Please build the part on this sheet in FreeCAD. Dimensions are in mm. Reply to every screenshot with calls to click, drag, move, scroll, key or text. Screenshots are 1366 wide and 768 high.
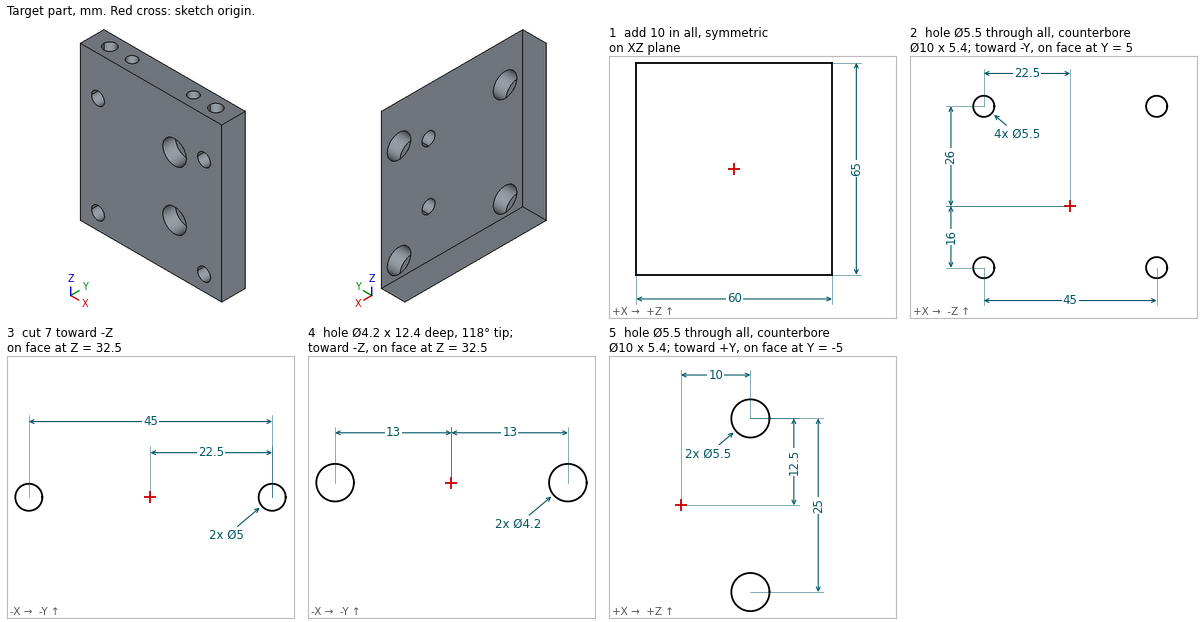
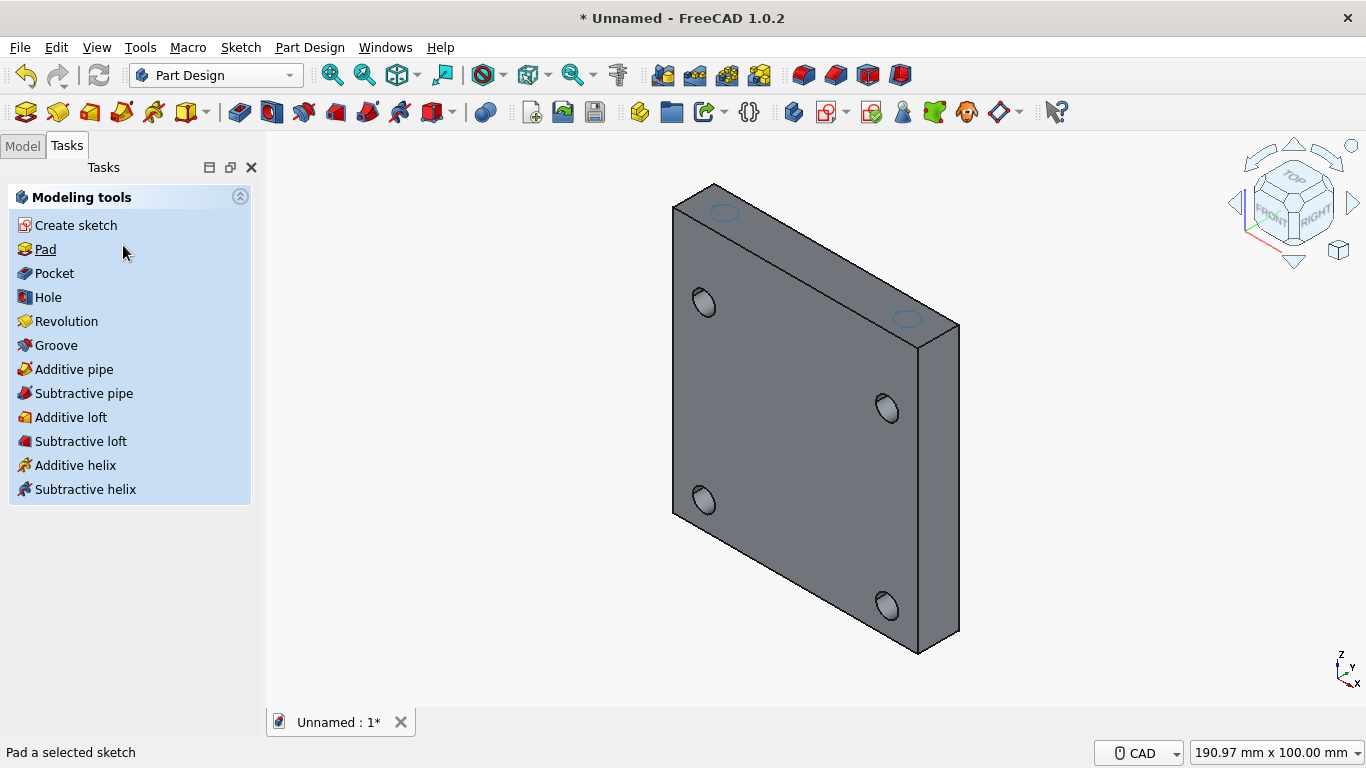
click(240, 112)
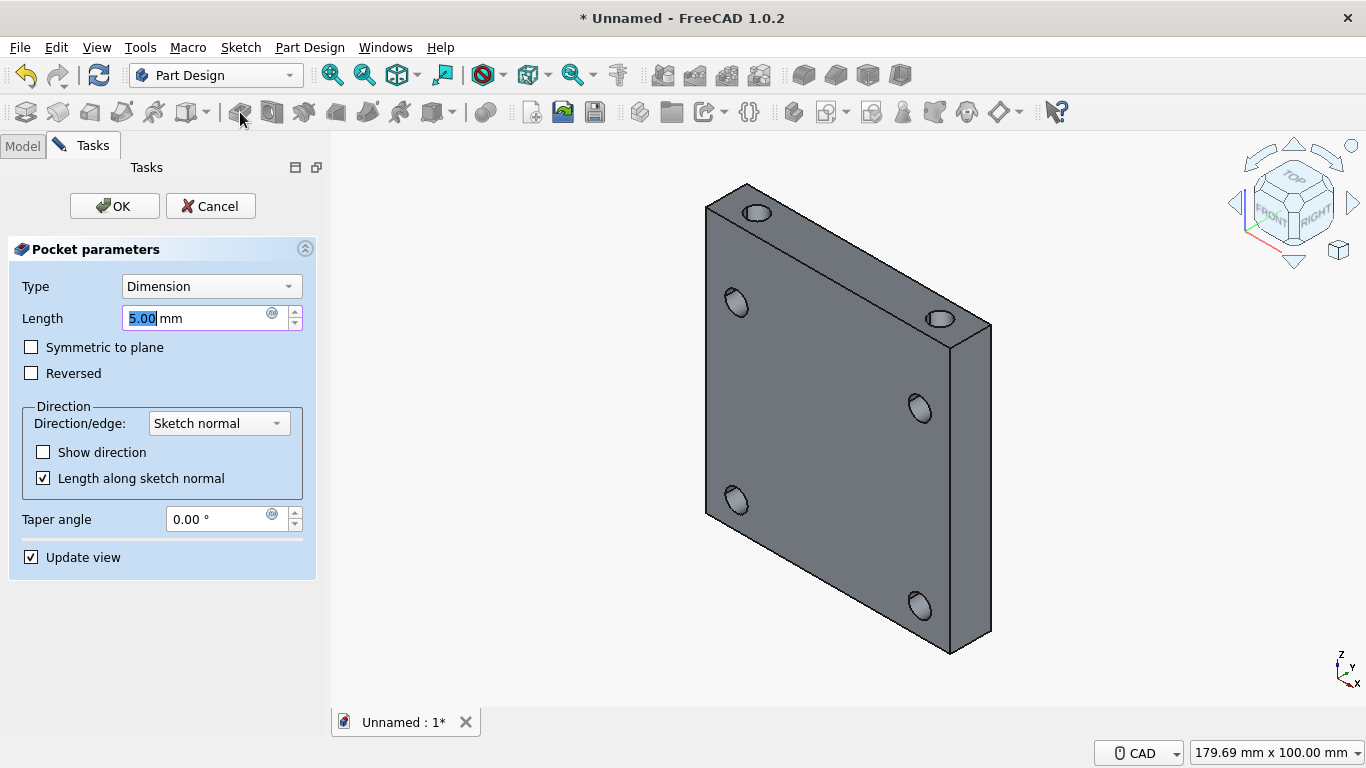
text(7)
key(Tab)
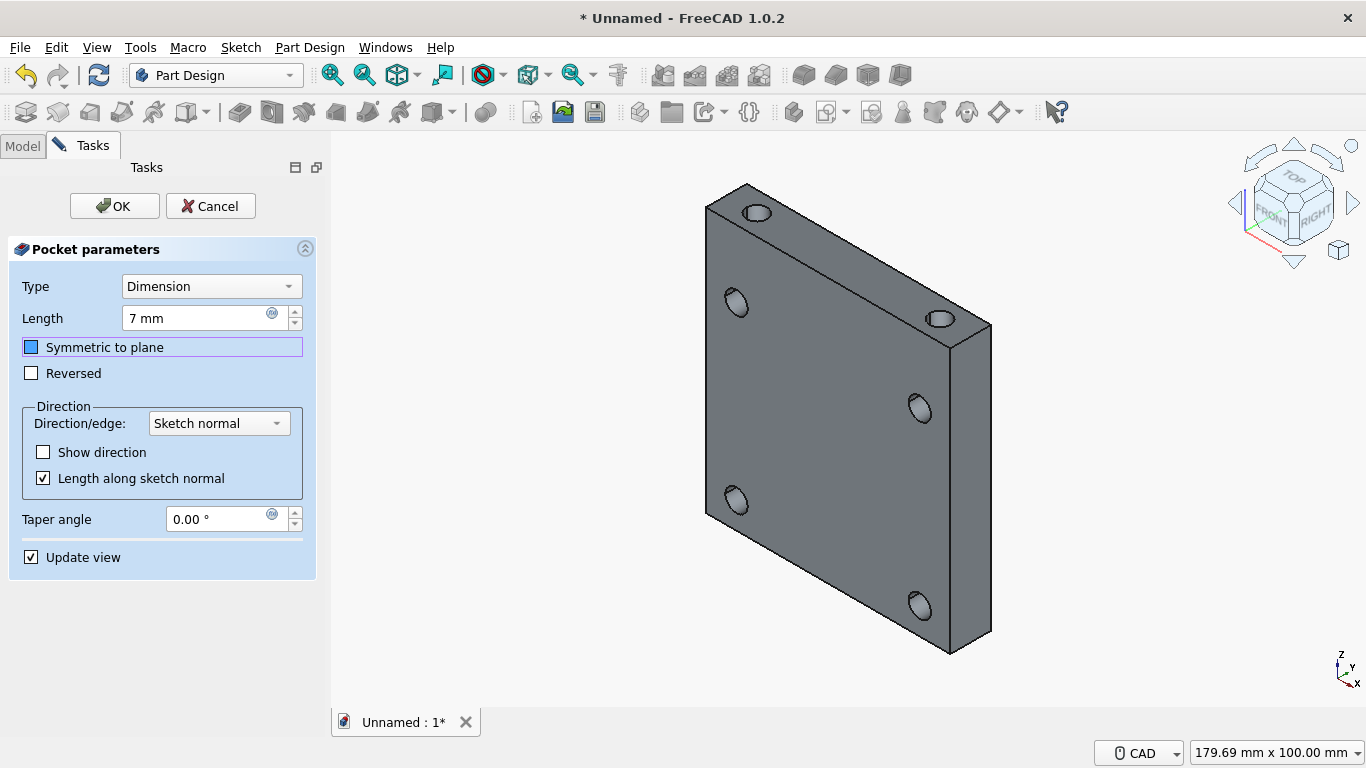
click(115, 206)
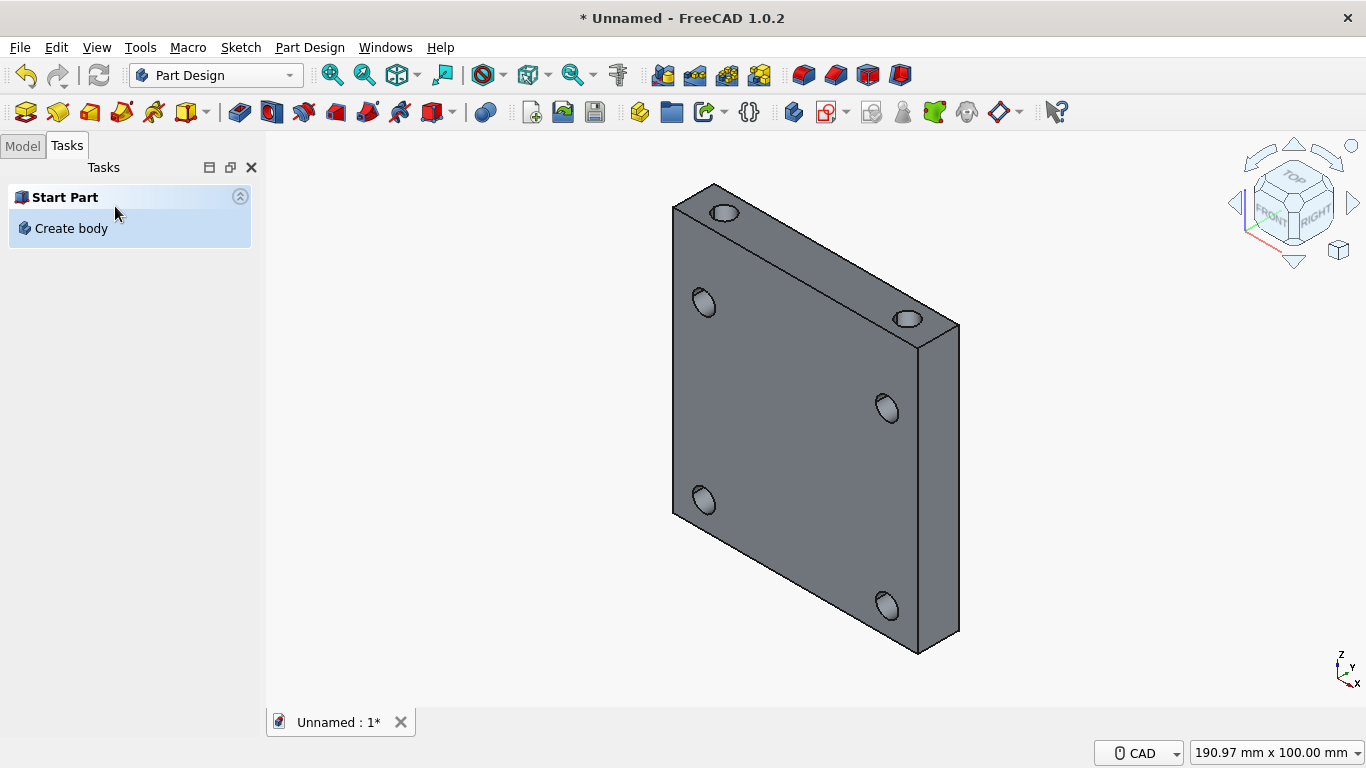
click(851, 285)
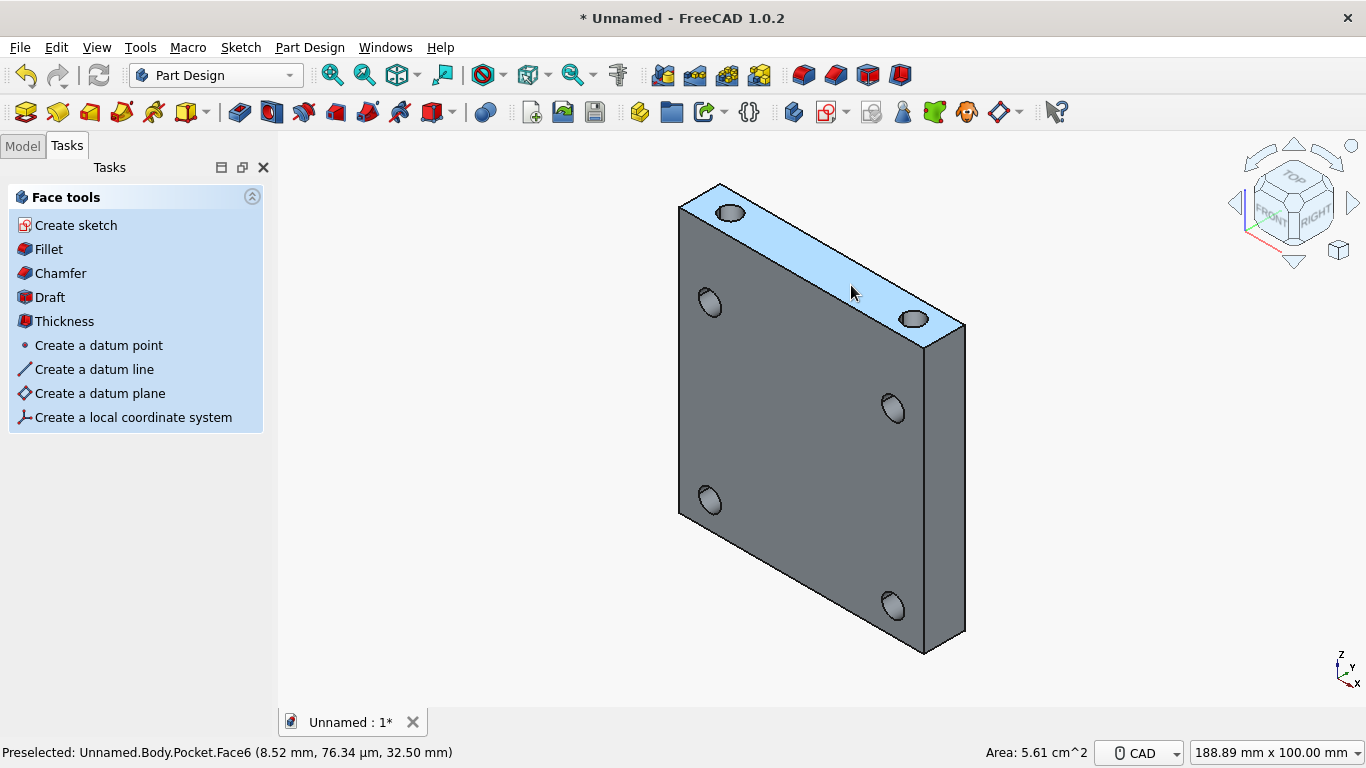
click(826, 112)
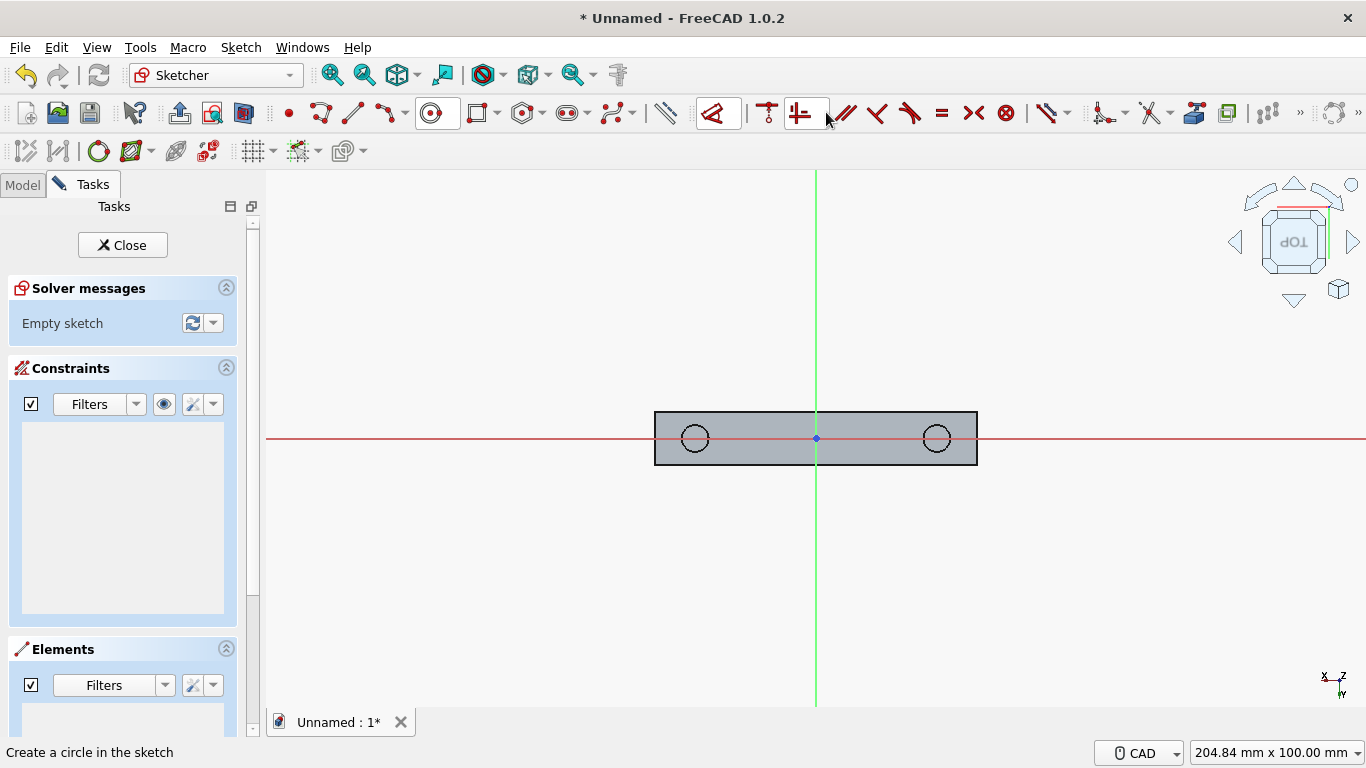
scroll(838, 439, up, 7)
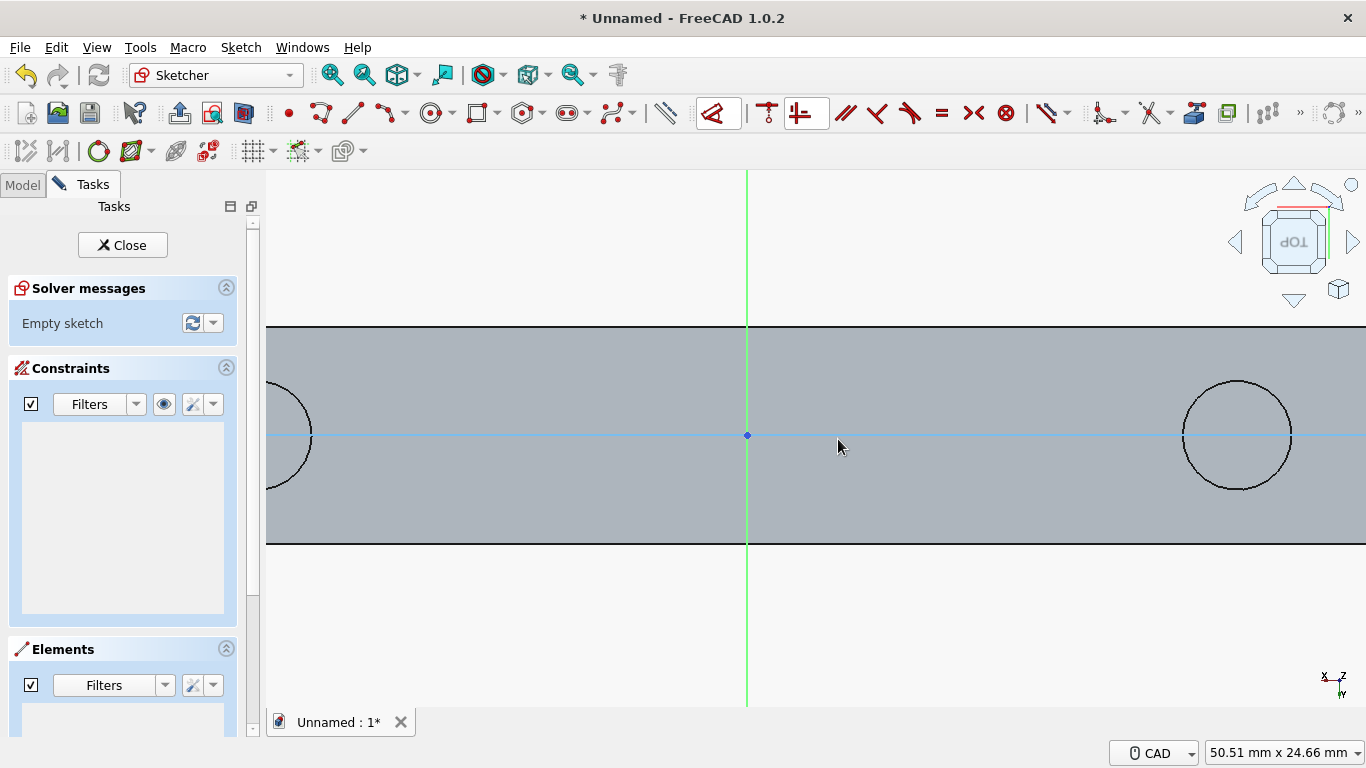
key(g)
key(c)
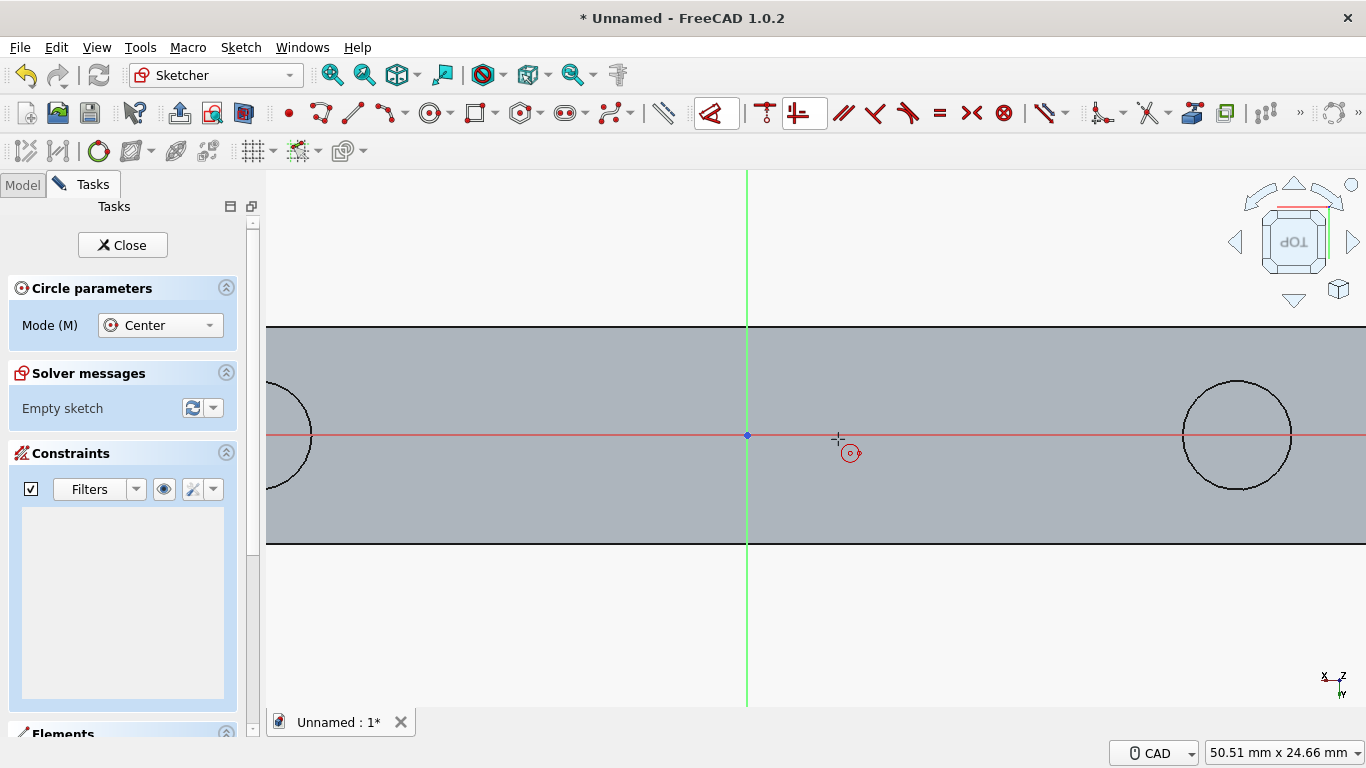
click(1030, 435)
click(1063, 403)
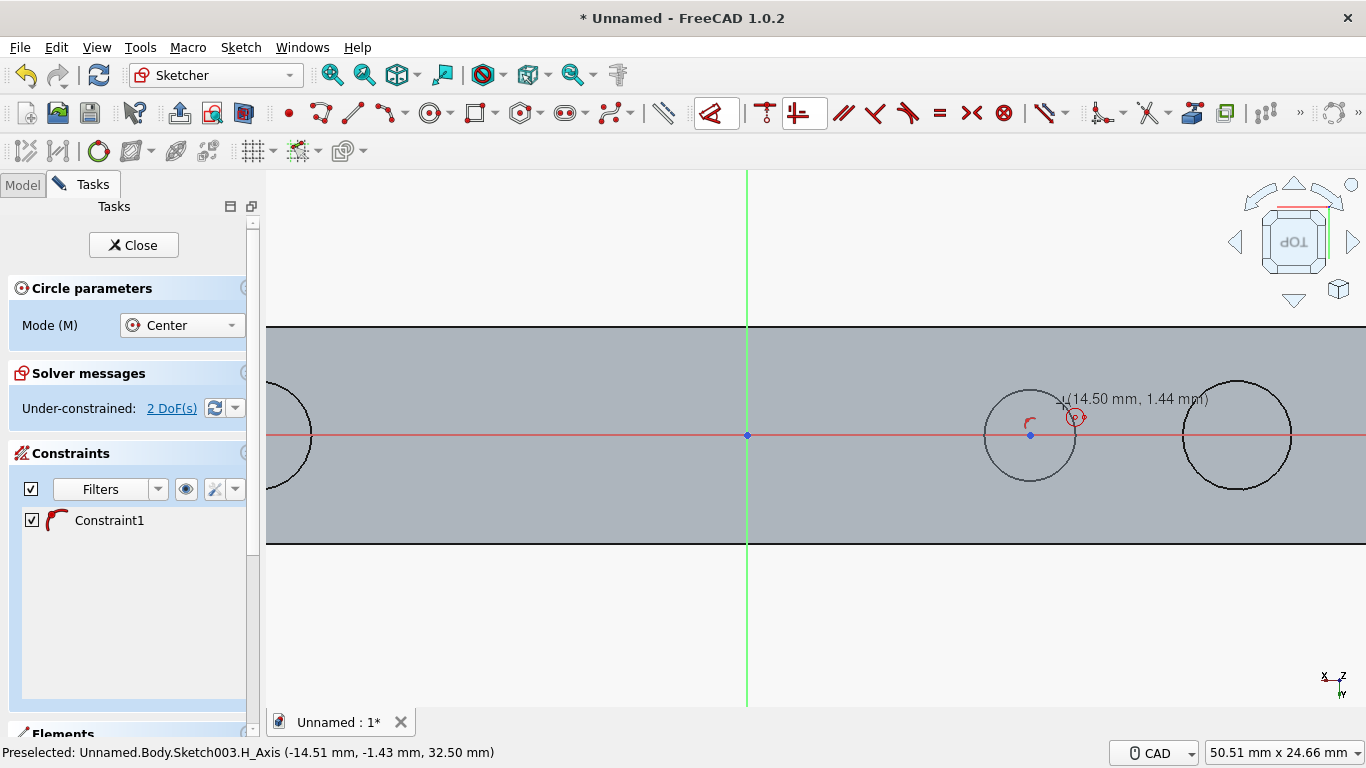
click(464, 435)
click(496, 403)
key(Escape)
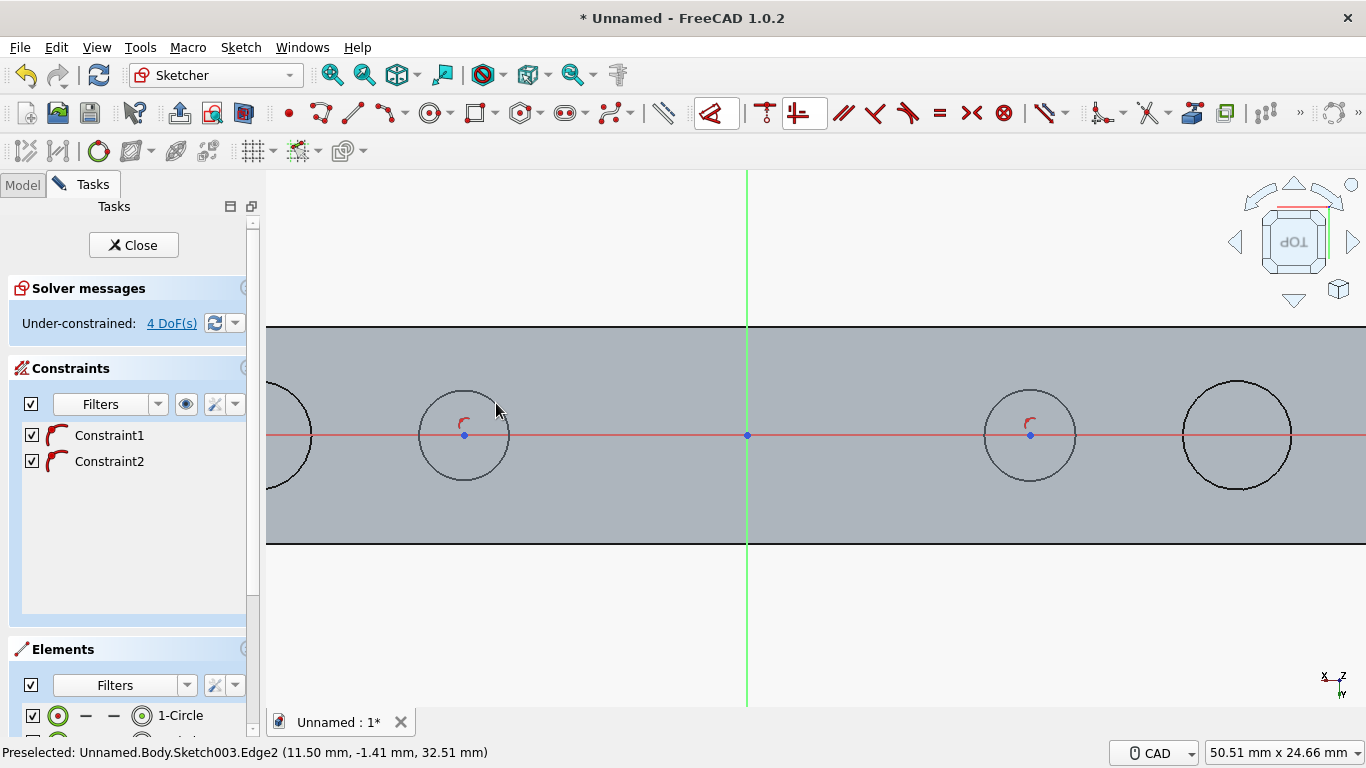
click(1062, 403)